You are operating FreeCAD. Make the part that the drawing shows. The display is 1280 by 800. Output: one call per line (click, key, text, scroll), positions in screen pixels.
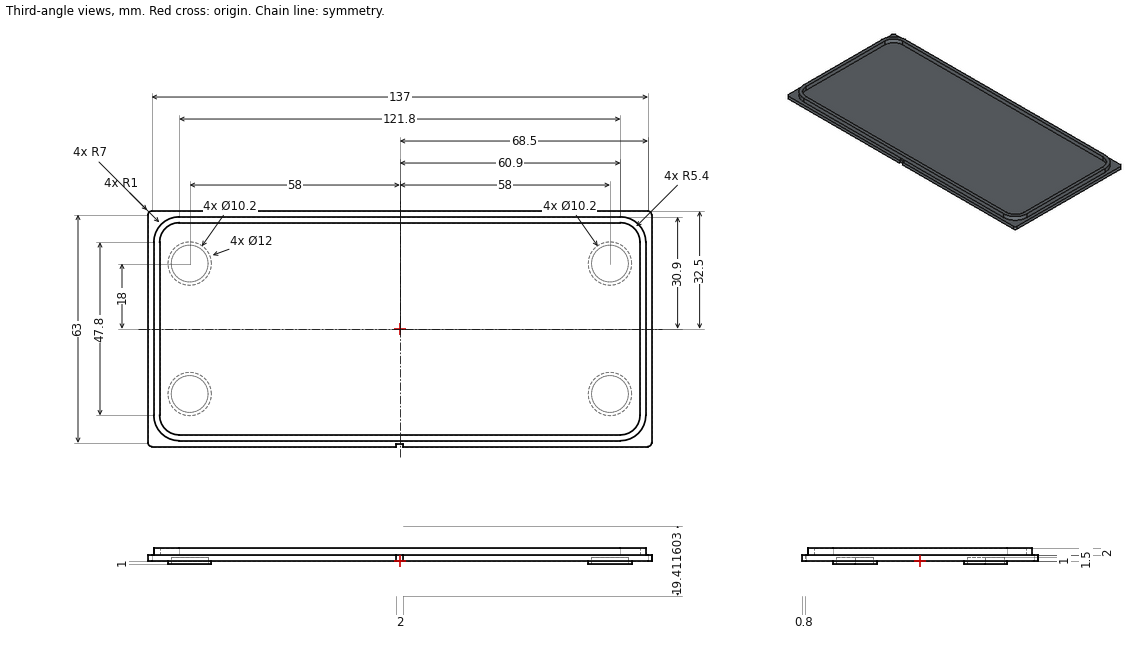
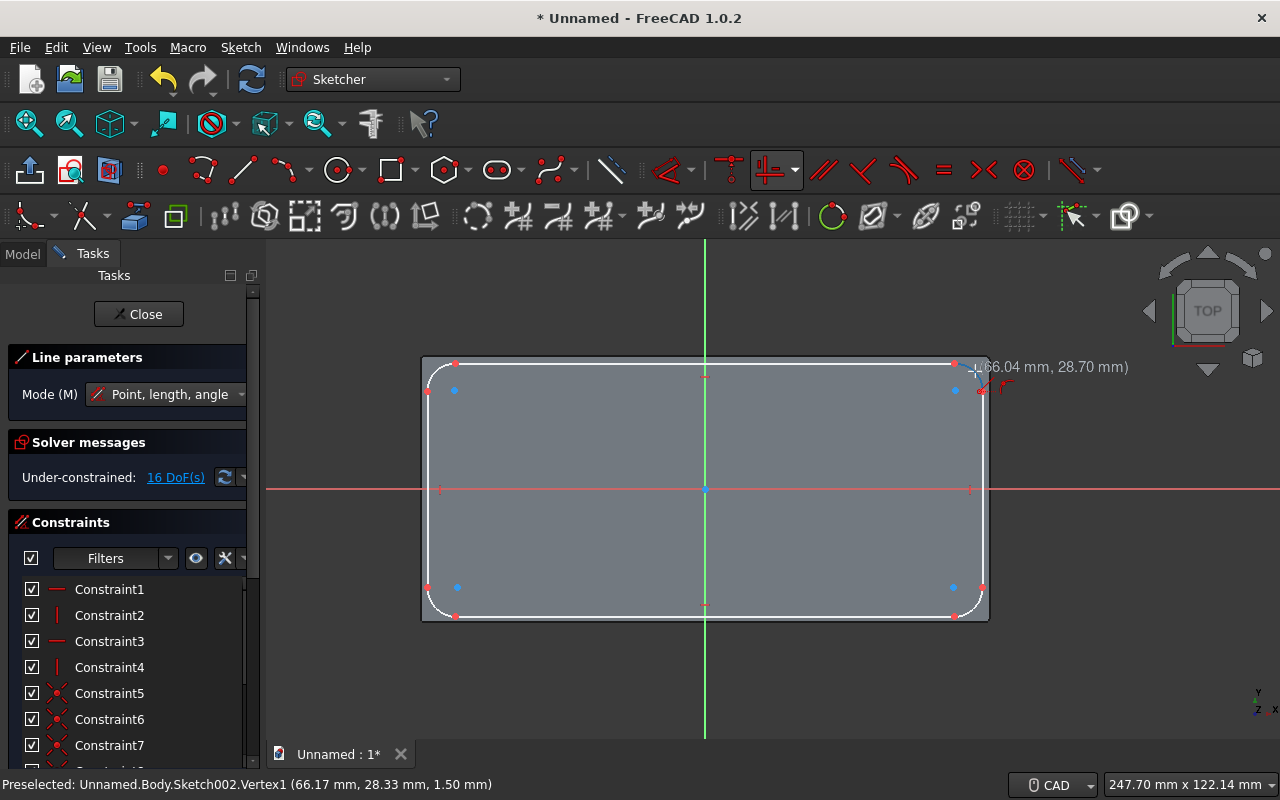
scroll(456, 369, up, 5)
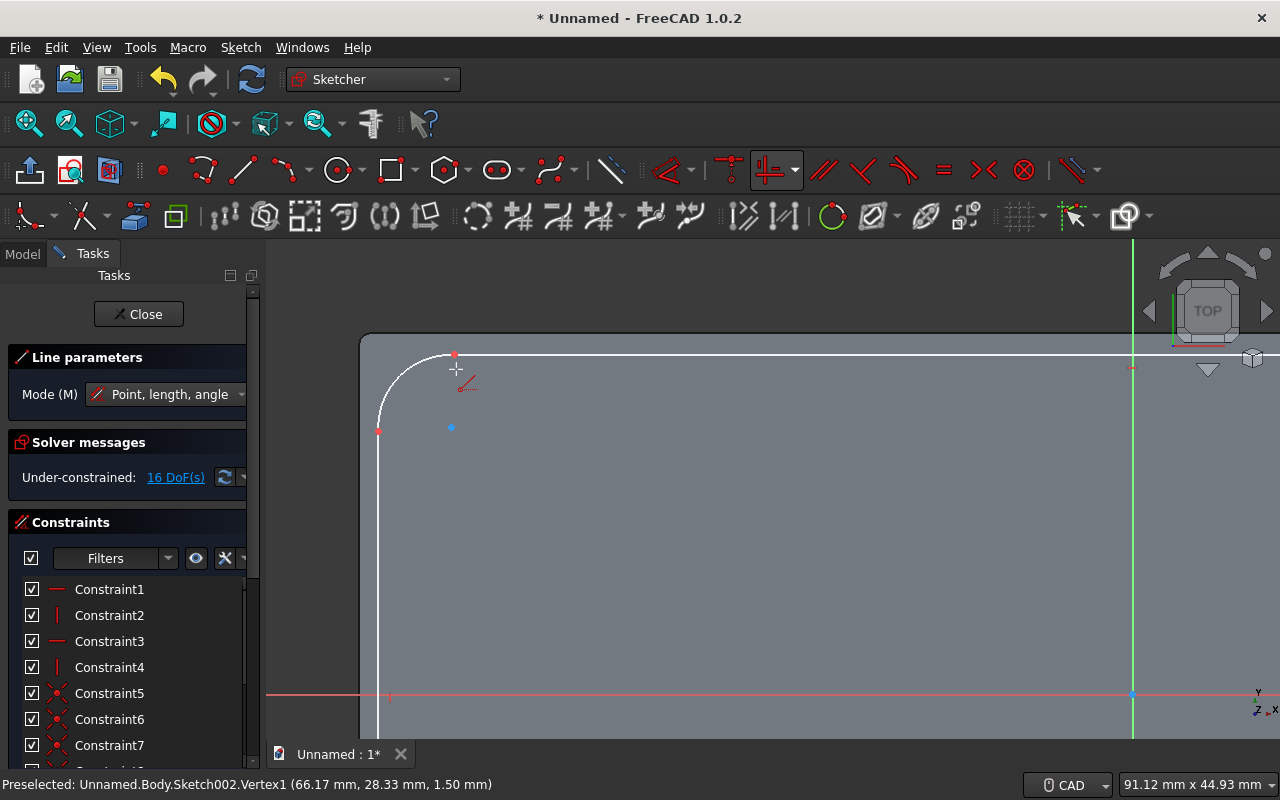
click(455, 369)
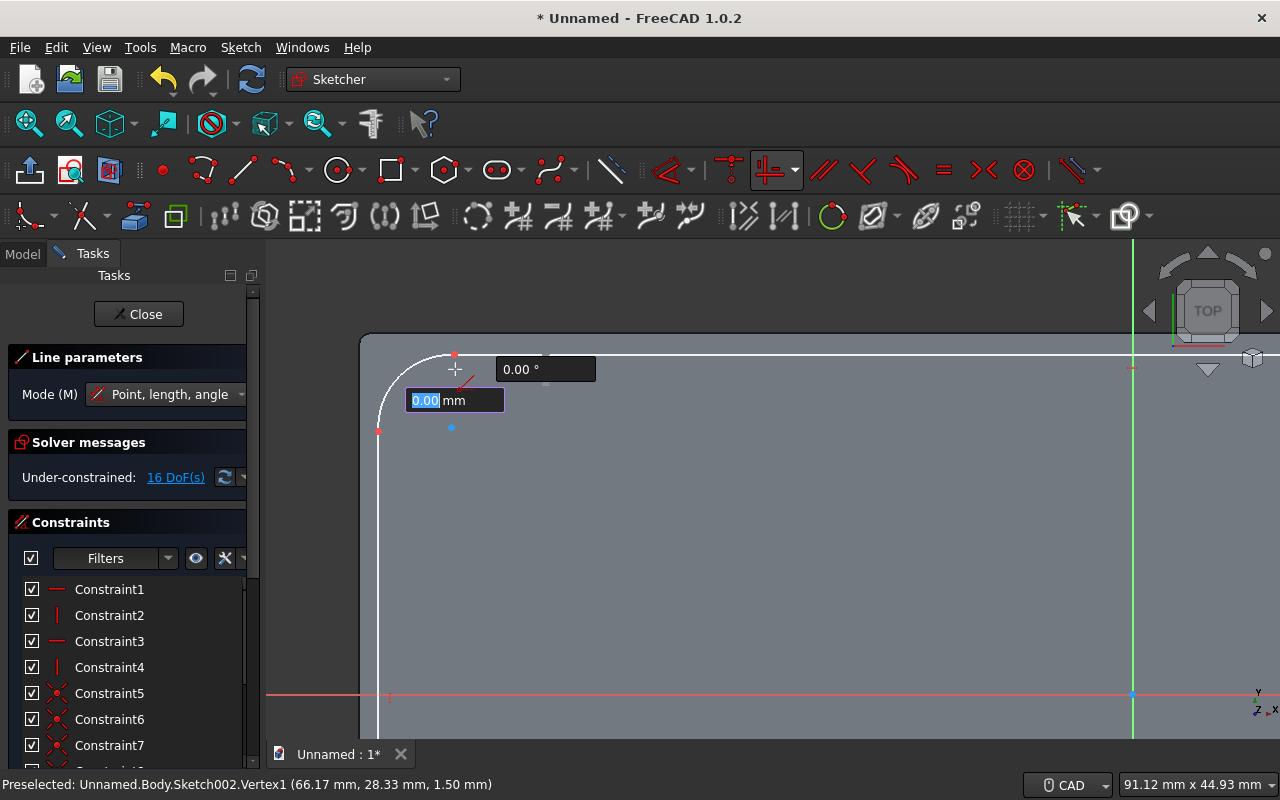
scroll(455, 369, down, 5)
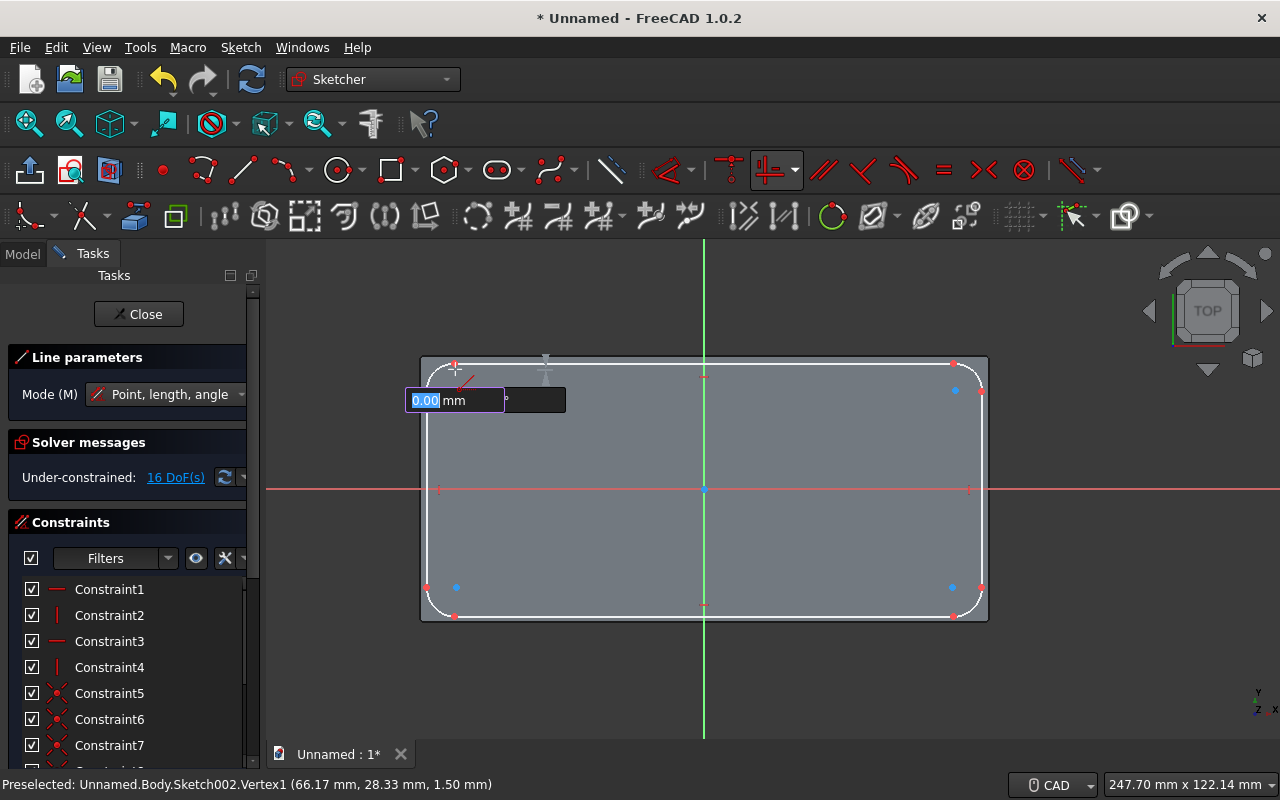
scroll(954, 369, up, 5)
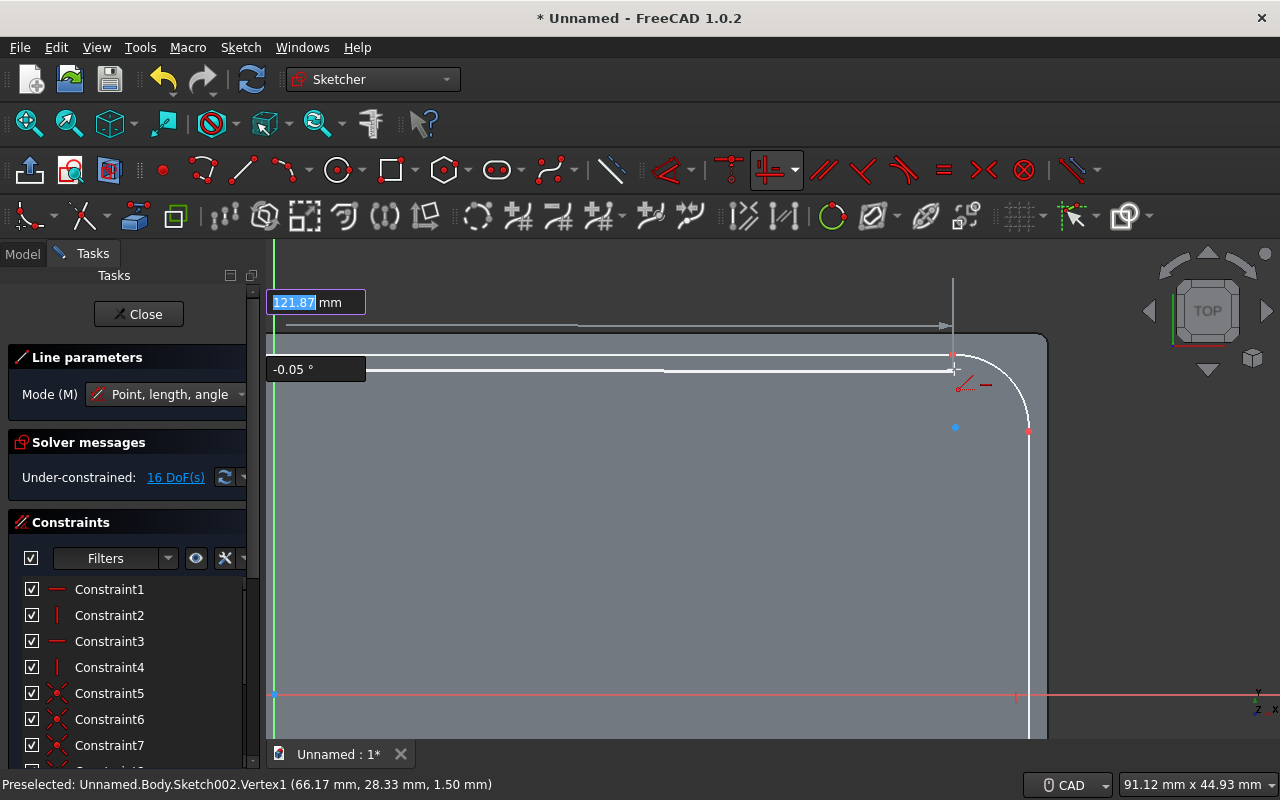
click(952, 369)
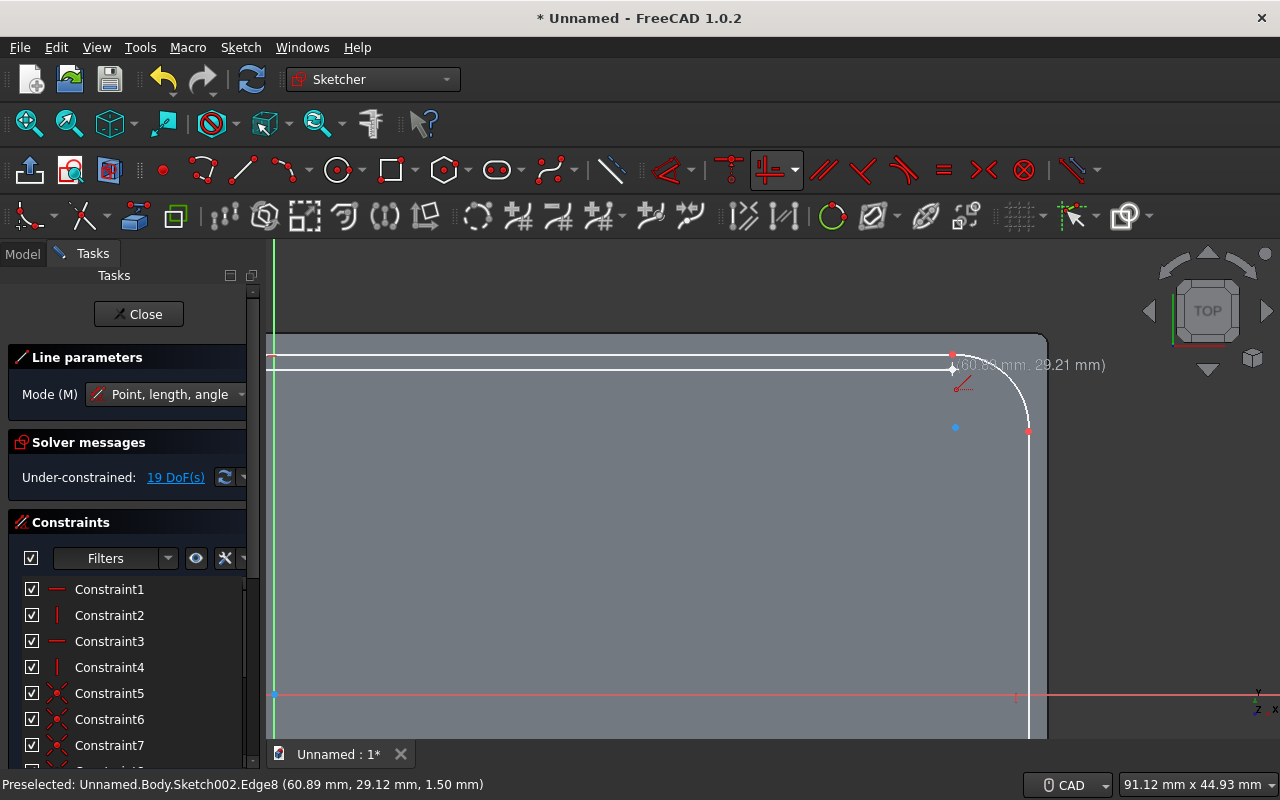
click(1012, 429)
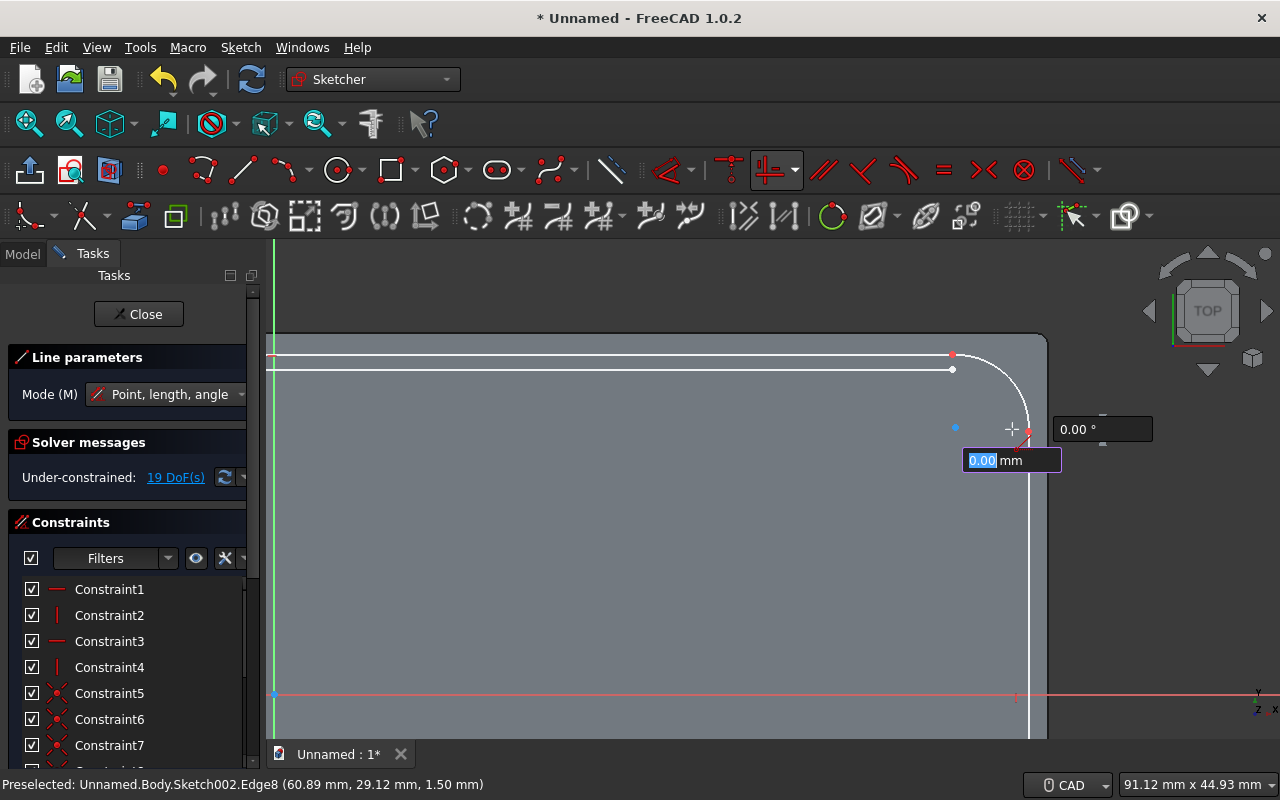
scroll(955, 369, down, 5)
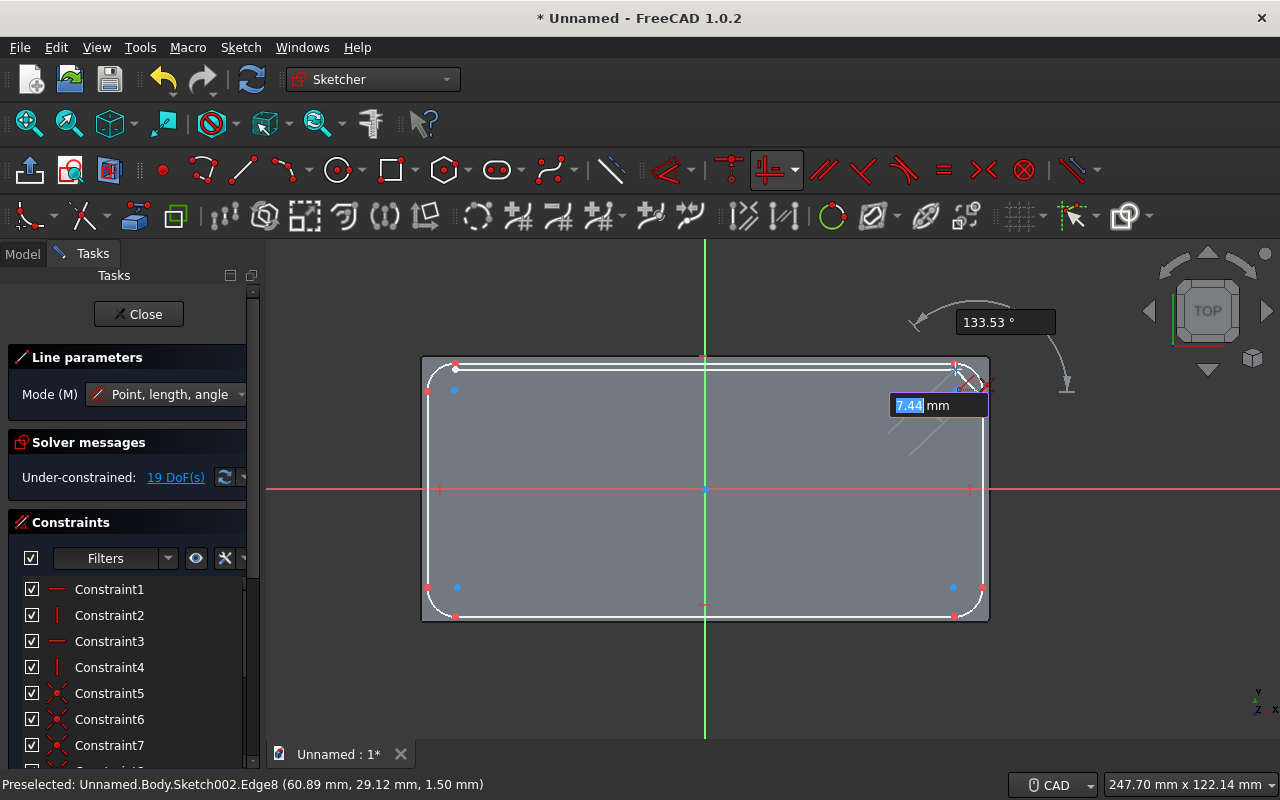
scroll(976, 587, up, 5)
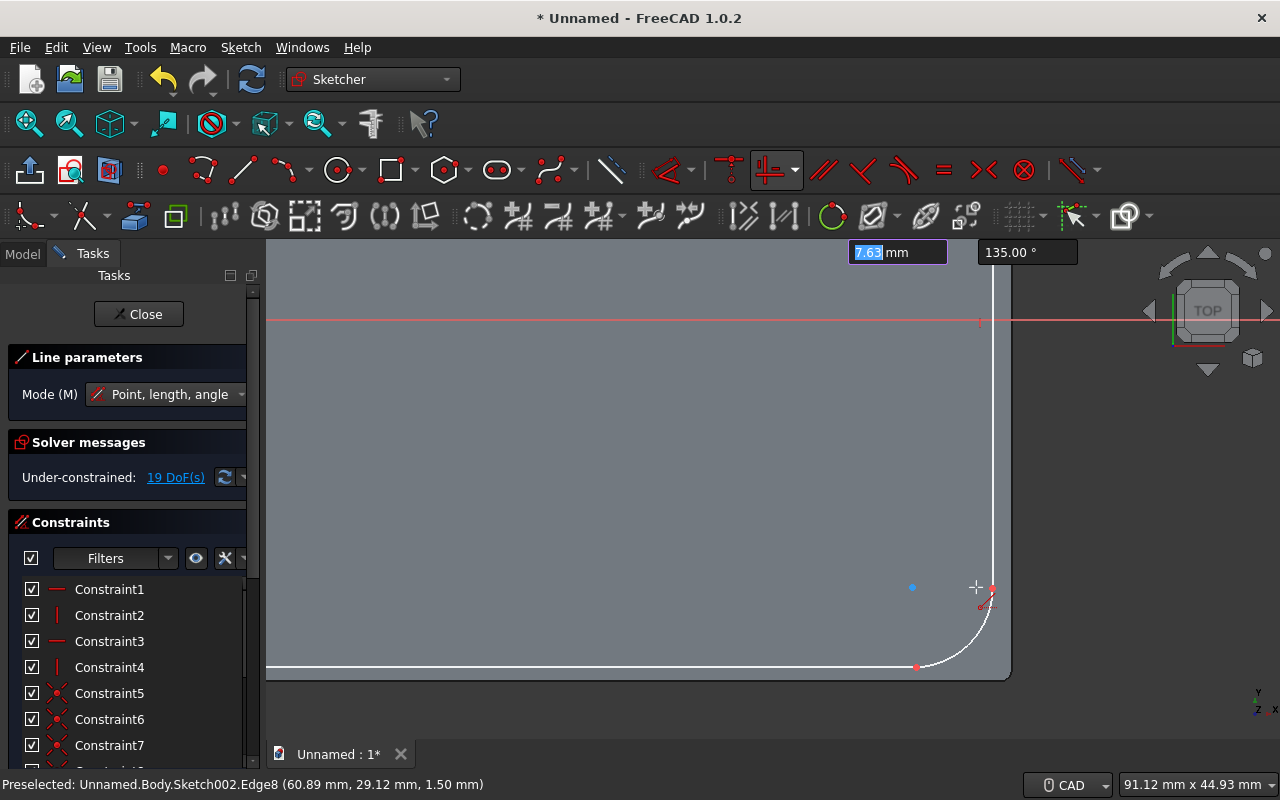
click(976, 586)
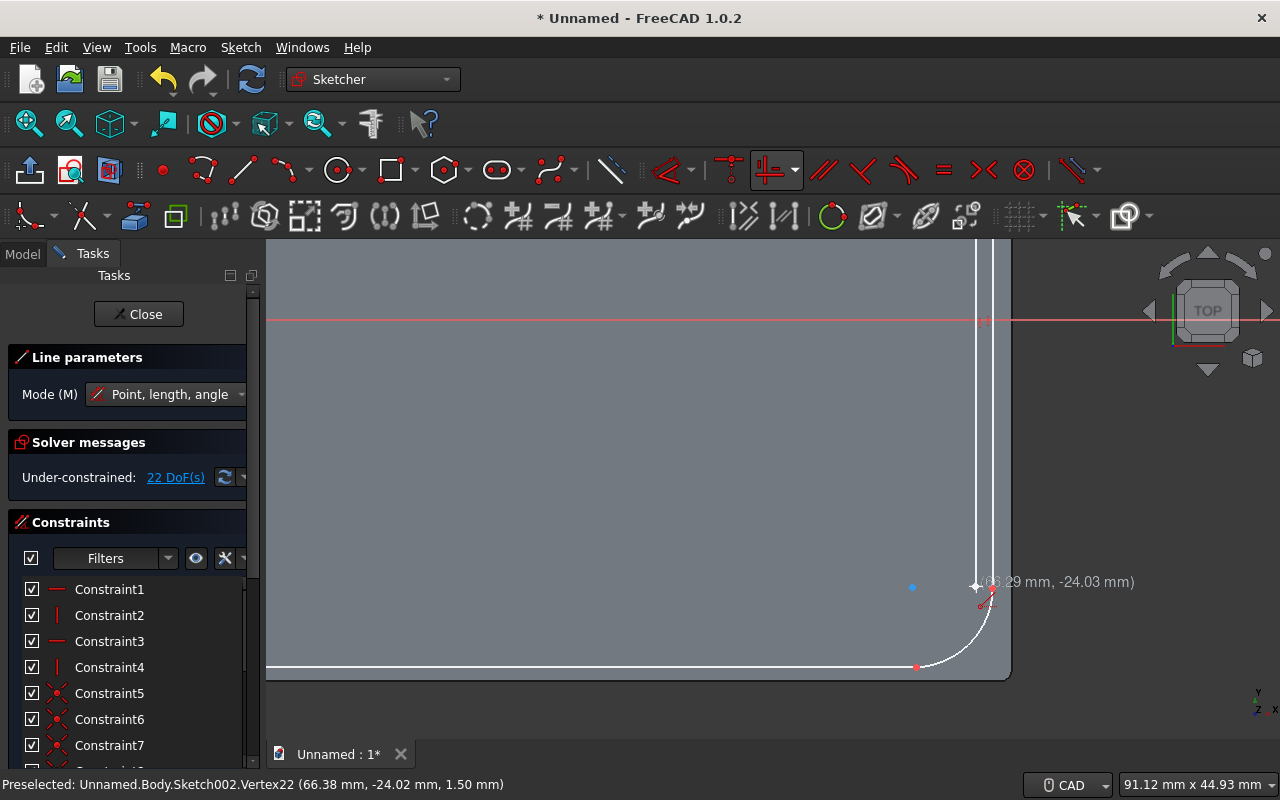
click(916, 646)